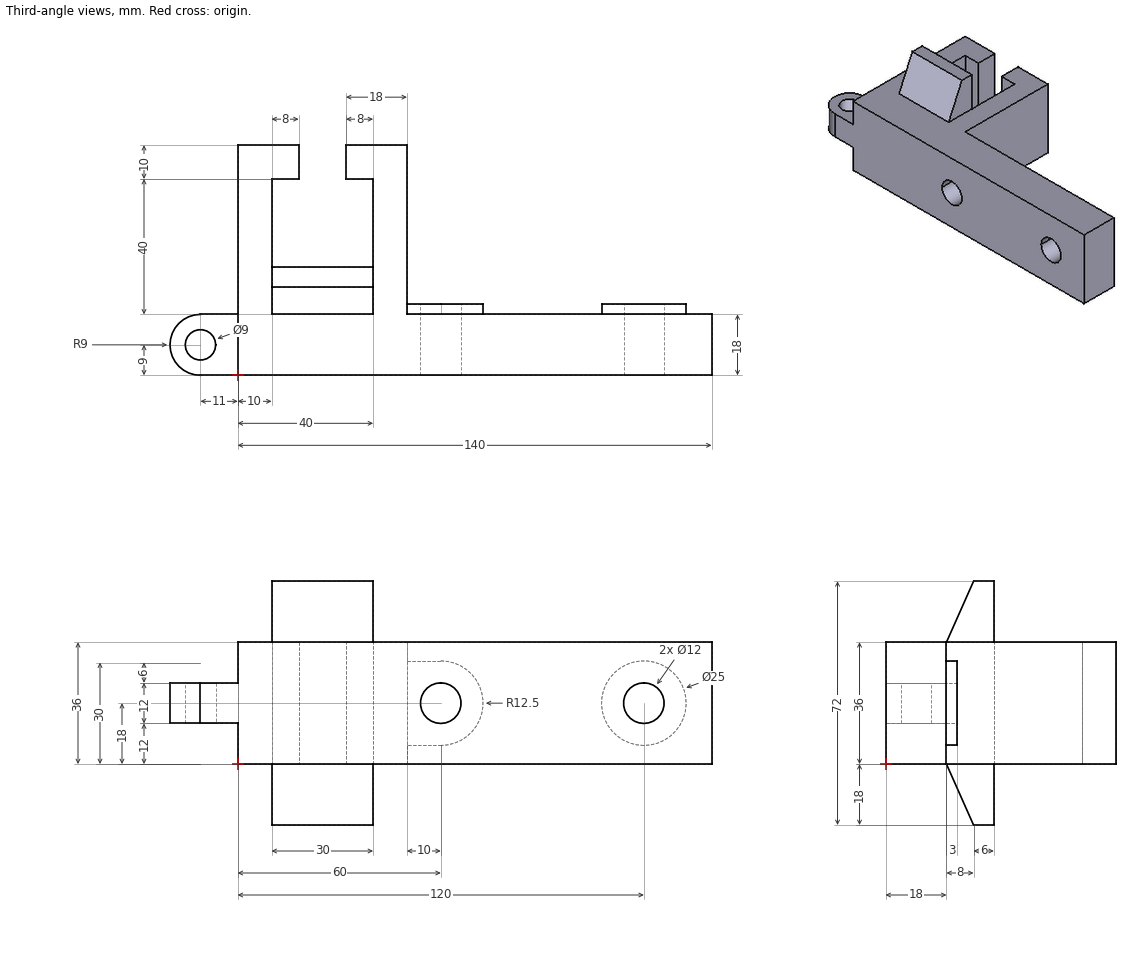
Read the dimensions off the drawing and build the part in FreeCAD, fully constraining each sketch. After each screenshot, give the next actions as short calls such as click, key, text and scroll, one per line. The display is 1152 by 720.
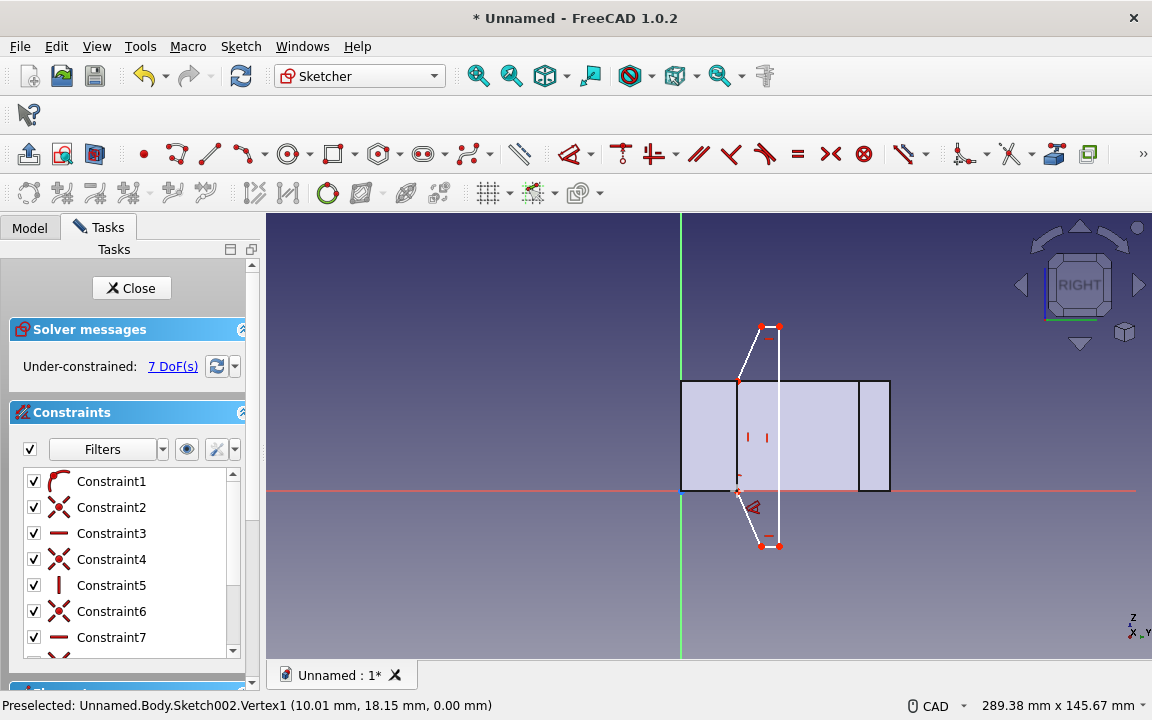
scroll(770, 547, up, 4)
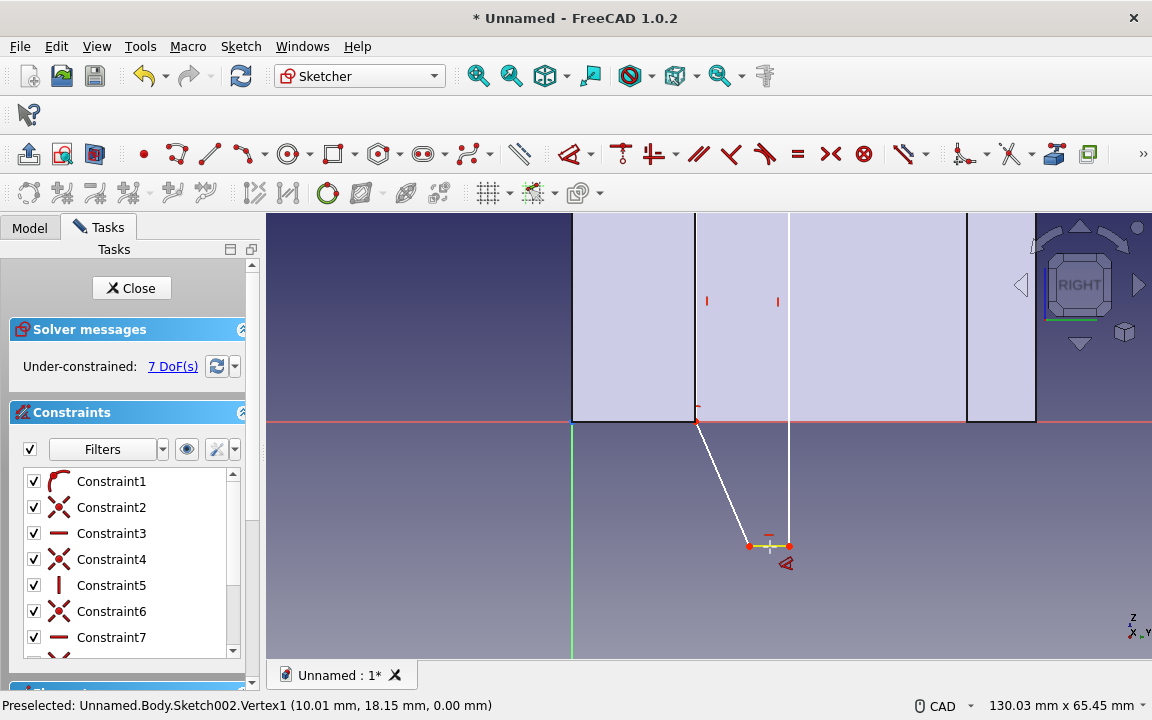
click(769, 546)
click(769, 580)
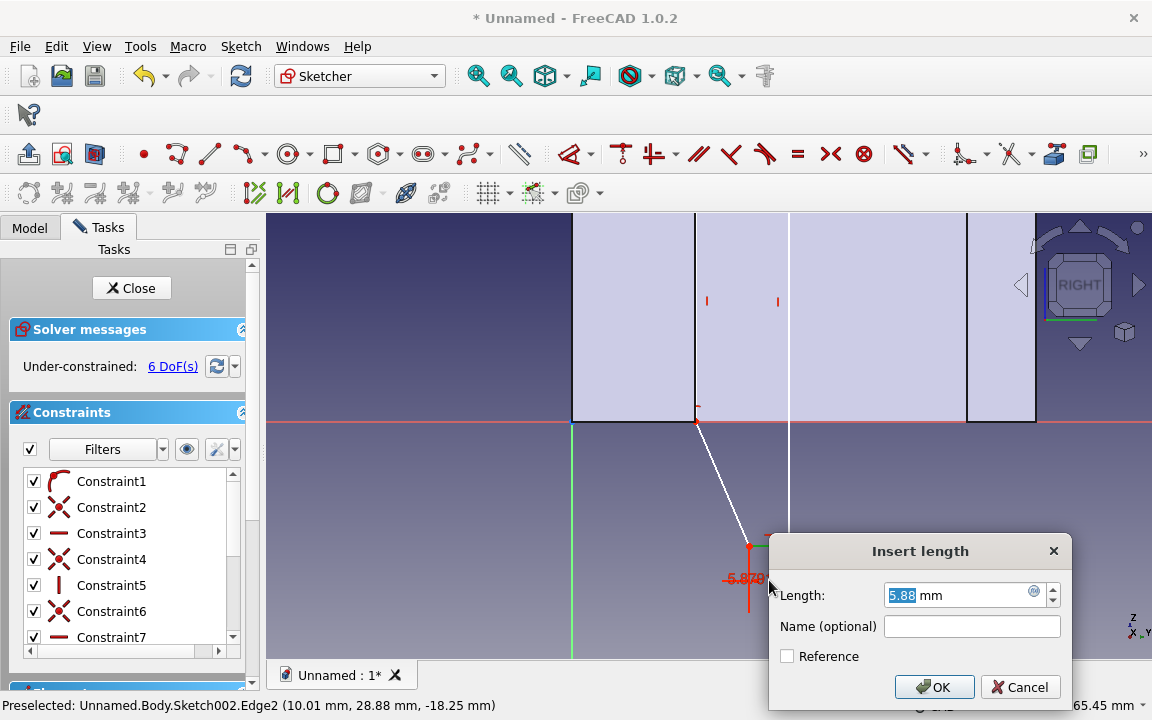
text(6)
key(Return)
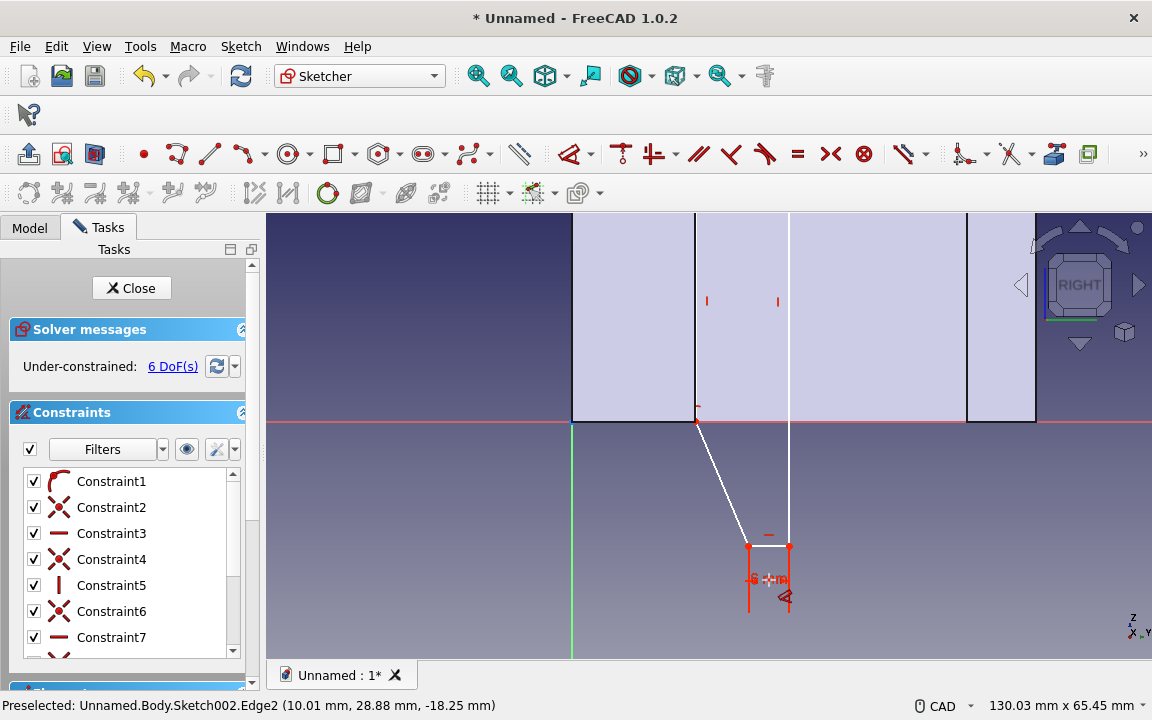
scroll(591, 603, down, 3)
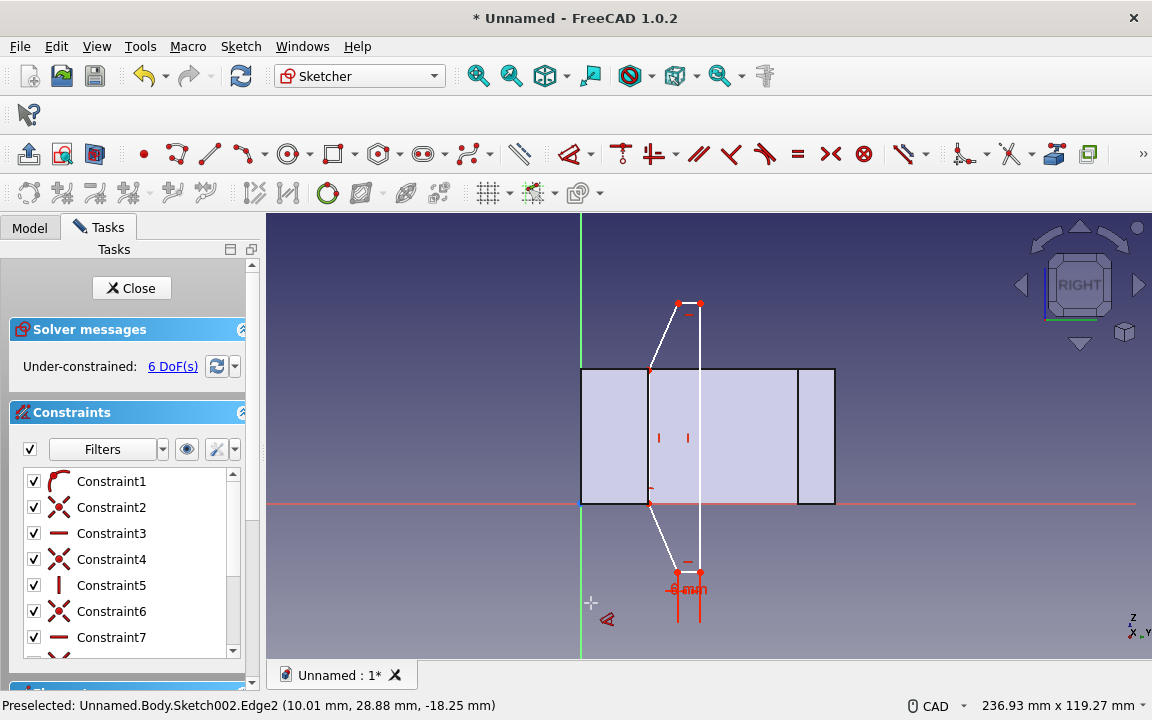
scroll(693, 303, up, 4)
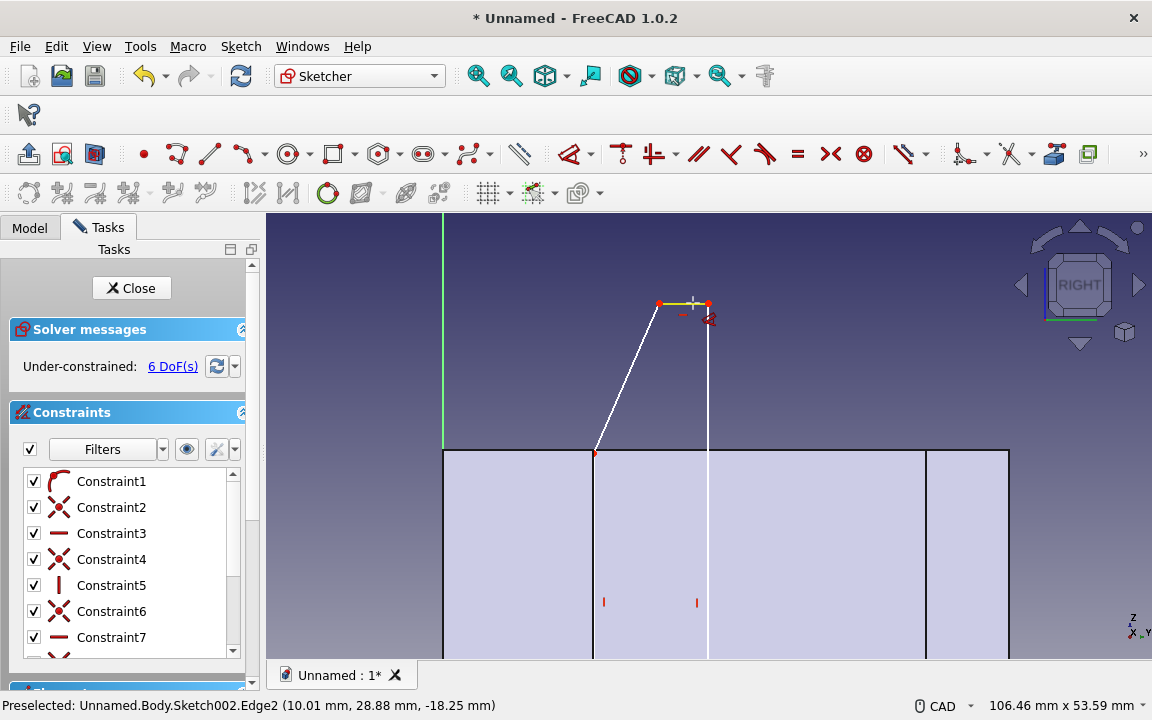
click(693, 304)
click(684, 270)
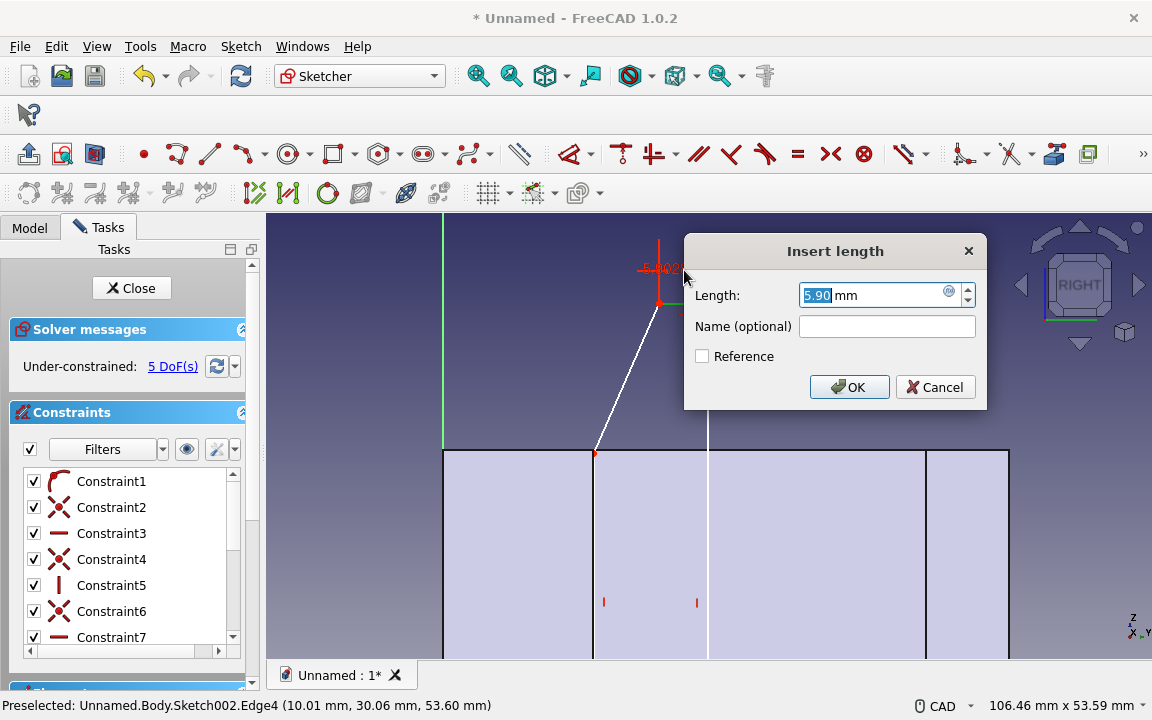
text(6)
key(Return)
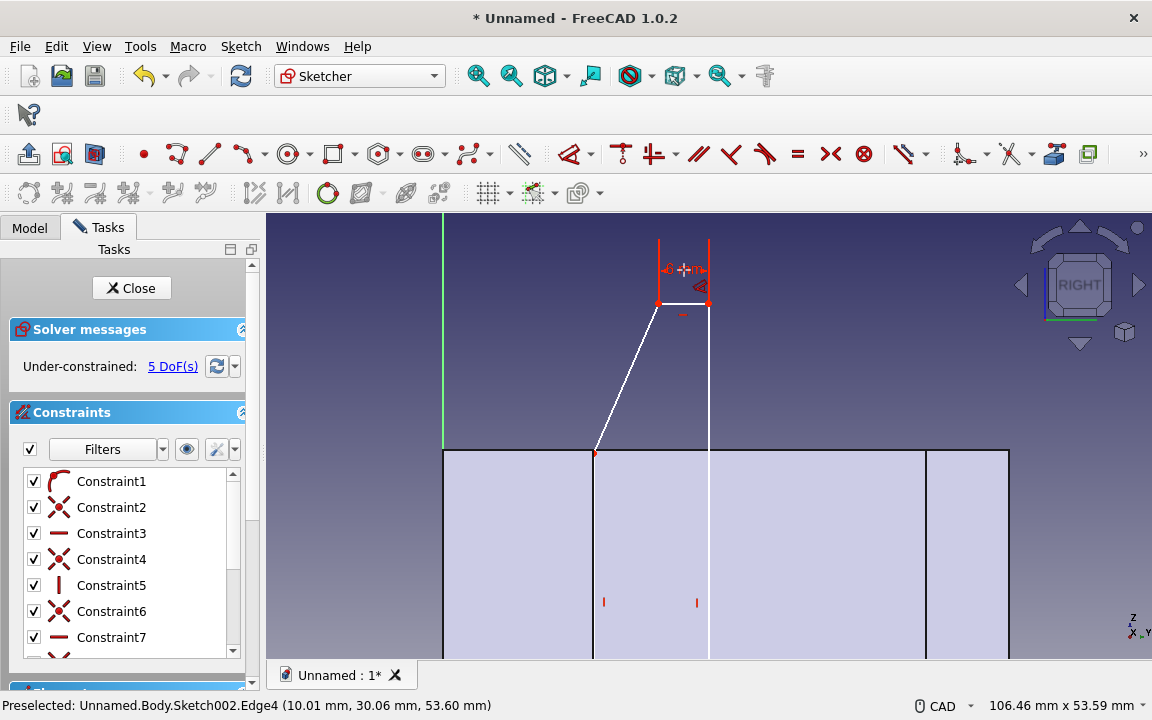
click(709, 483)
click(743, 467)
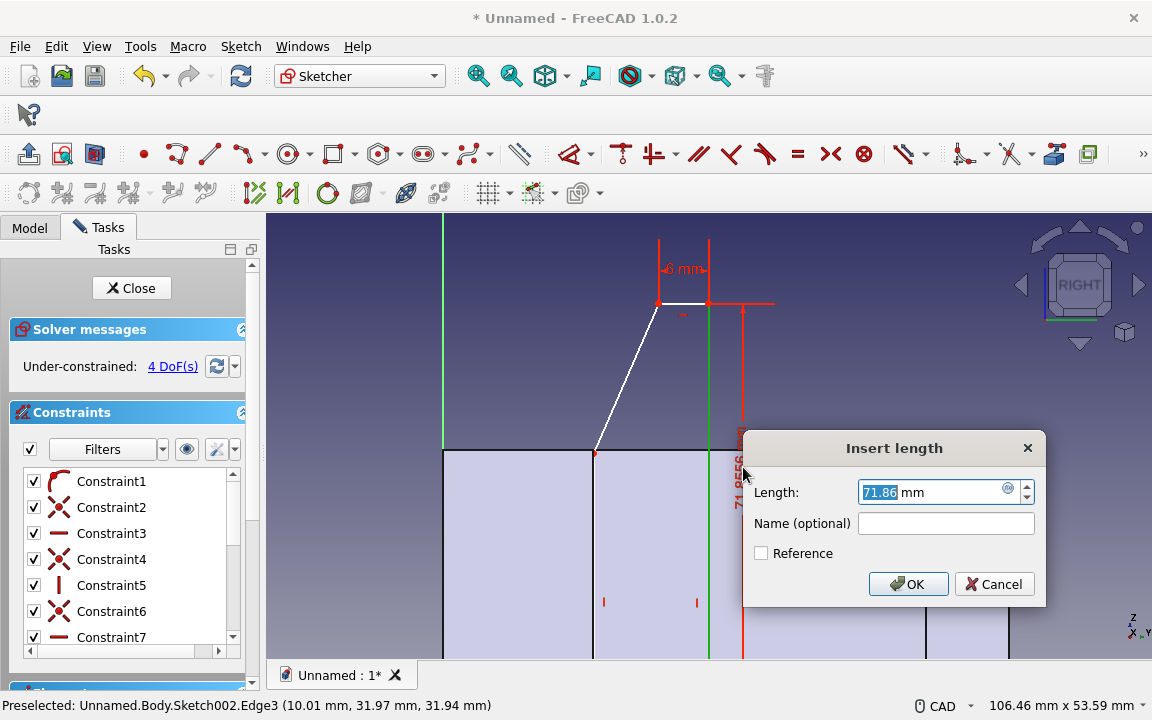
text(72)
key(Return)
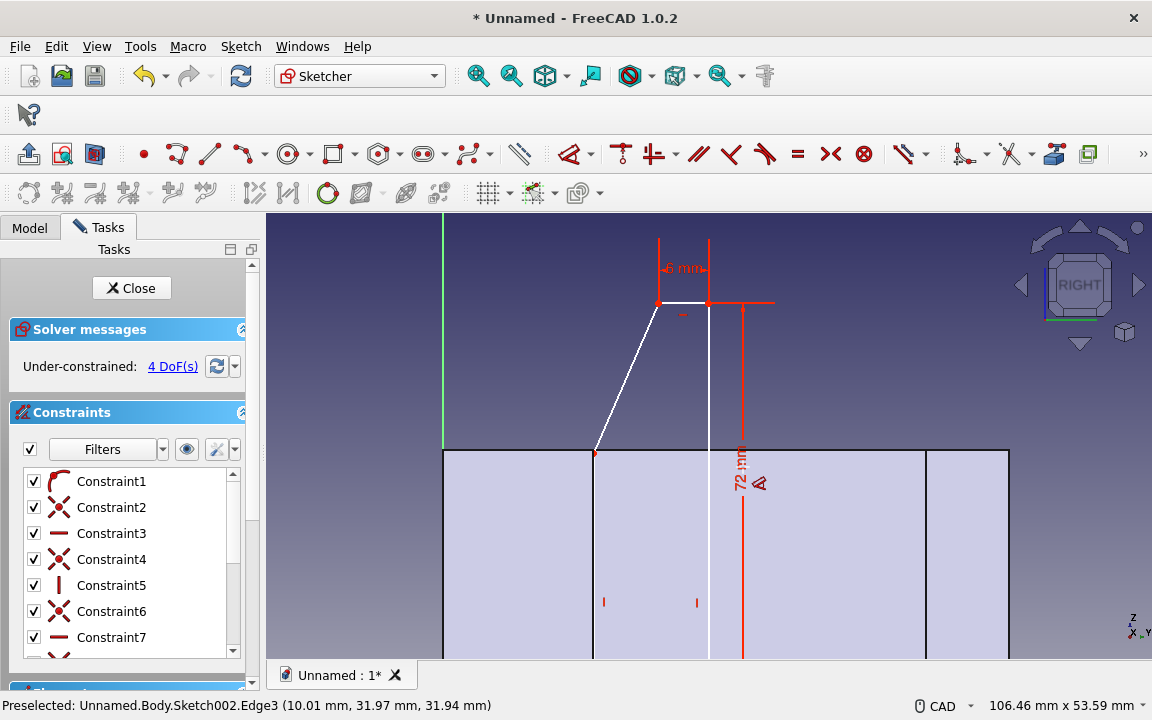
click(594, 542)
click(628, 542)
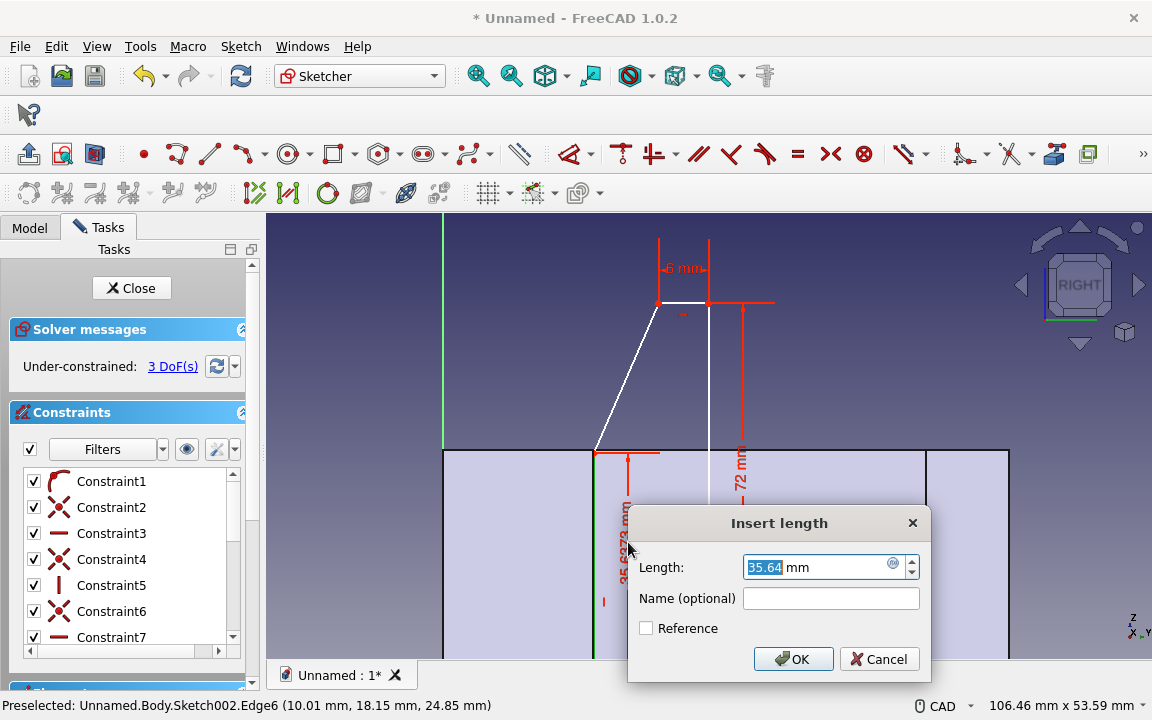
text(36)
key(Return)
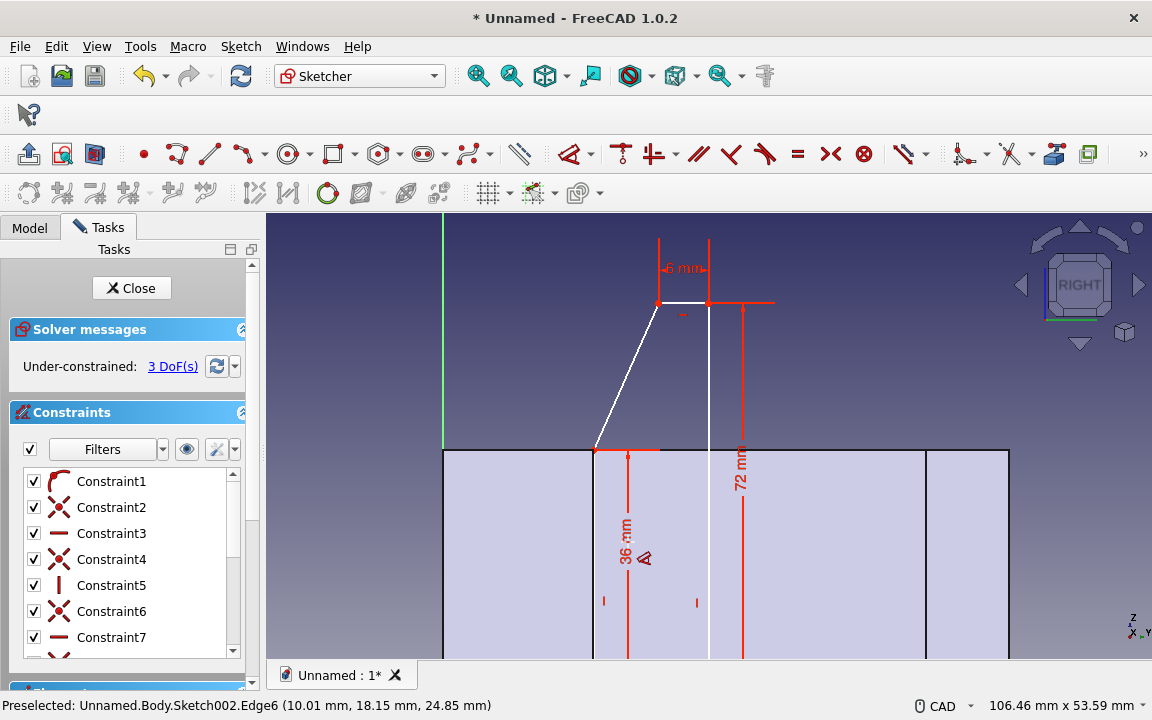
scroll(693, 302, down, 4)